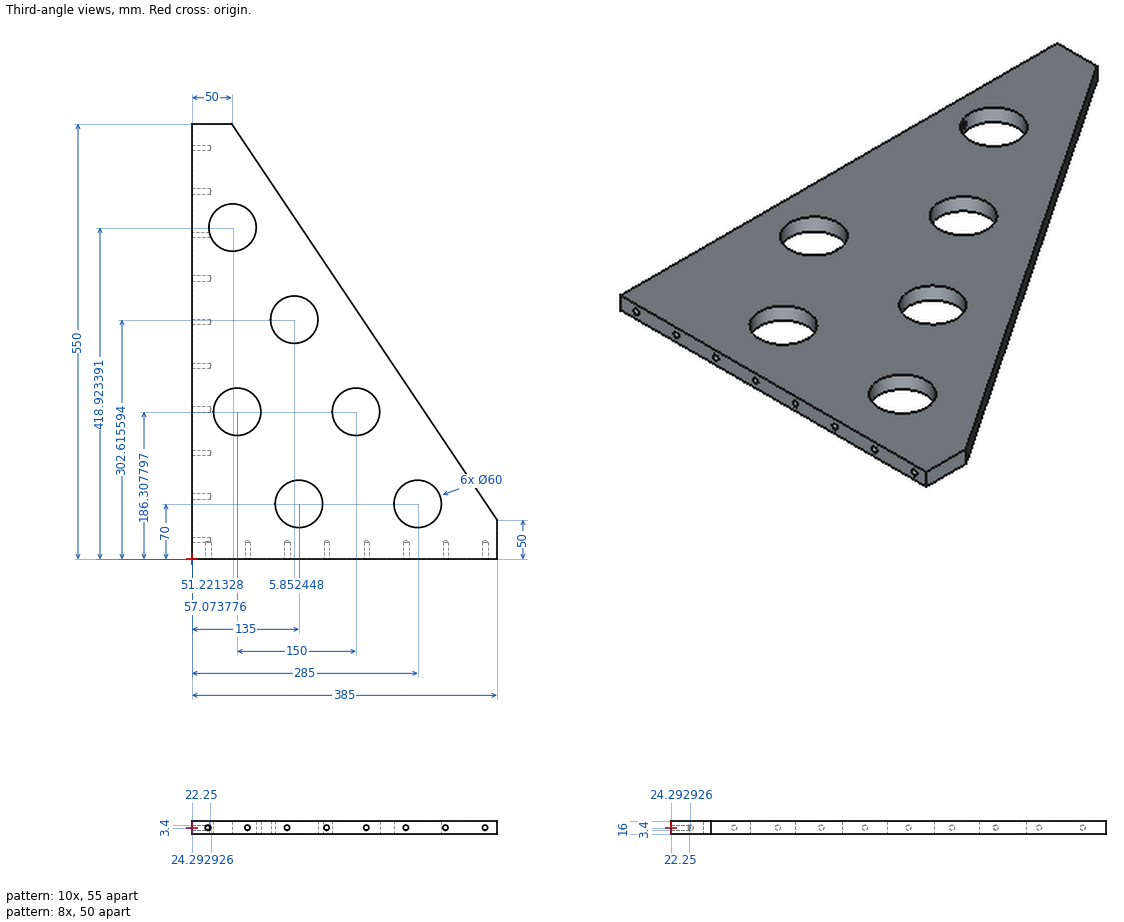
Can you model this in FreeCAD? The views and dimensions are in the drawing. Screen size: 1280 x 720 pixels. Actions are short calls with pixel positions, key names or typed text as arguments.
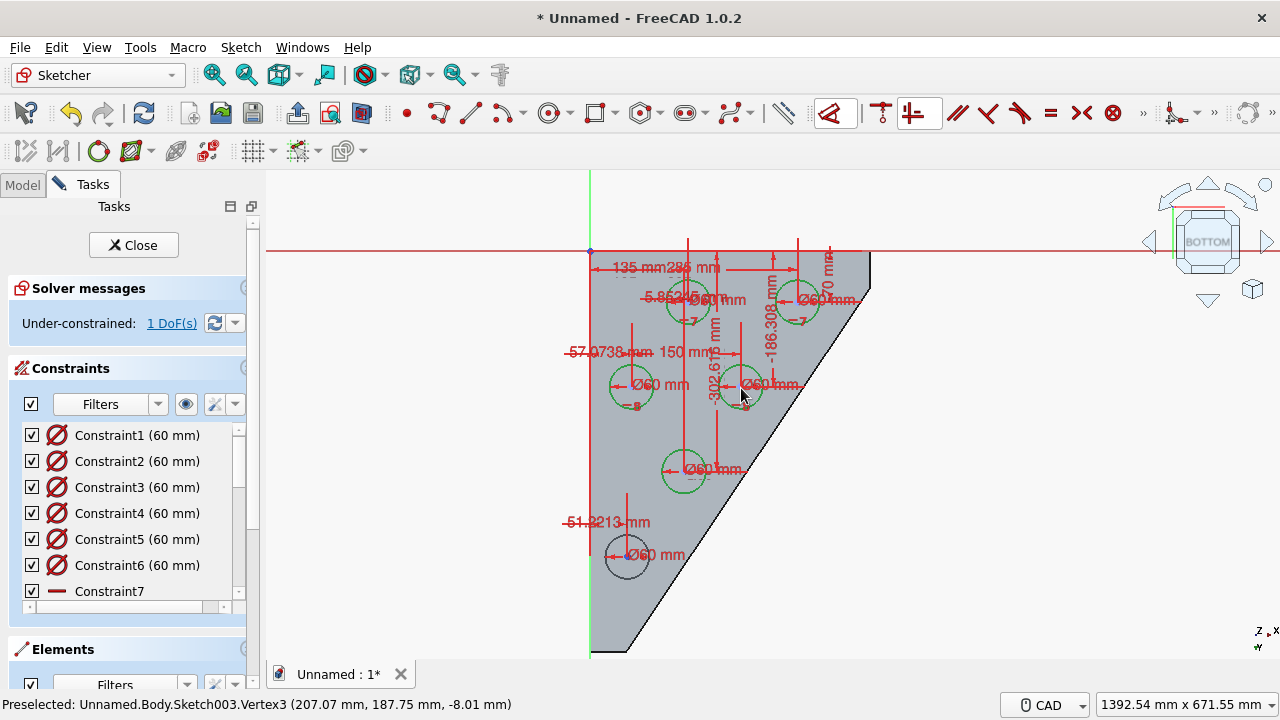
click(627, 557)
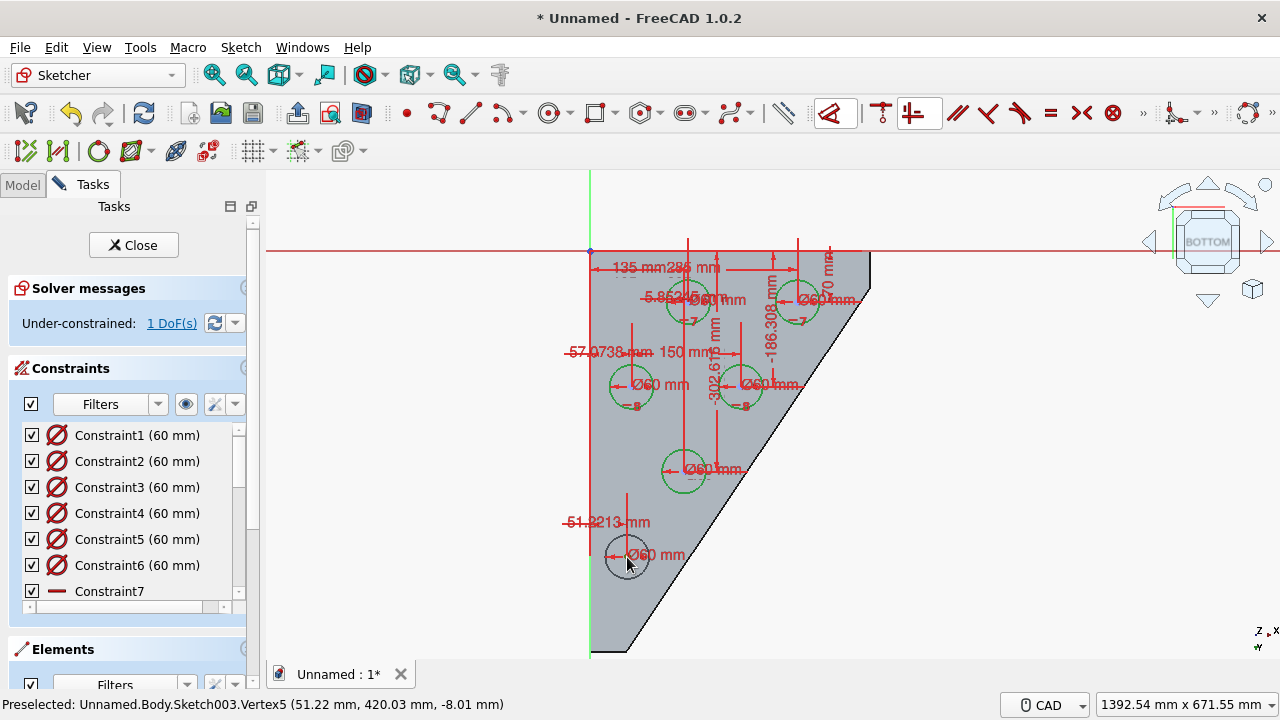
key(i)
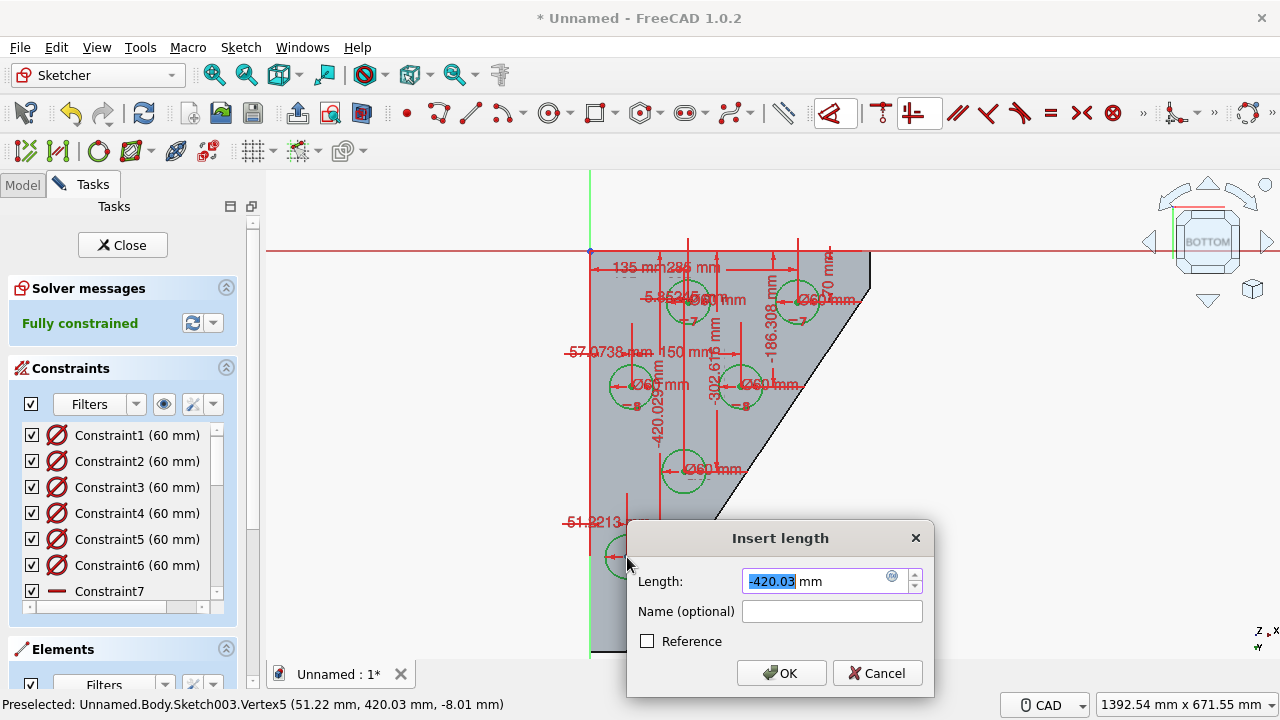
text(-418.923391)
key(Return)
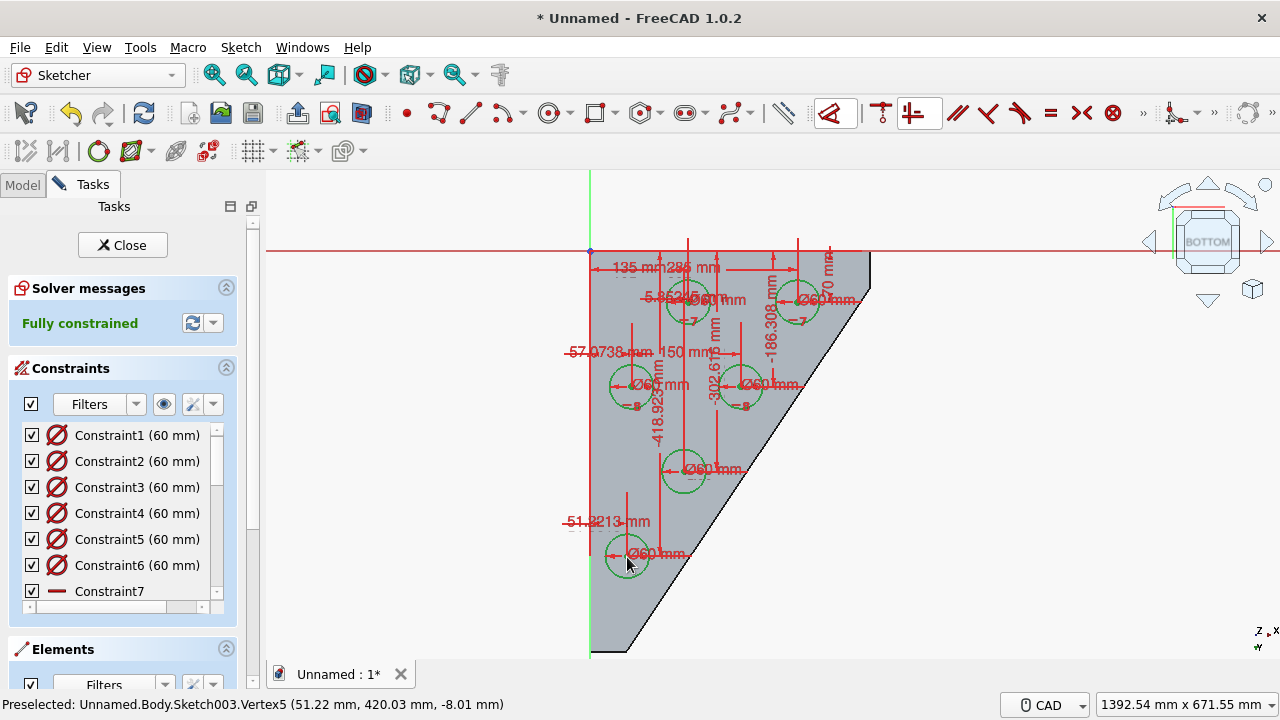
click(123, 245)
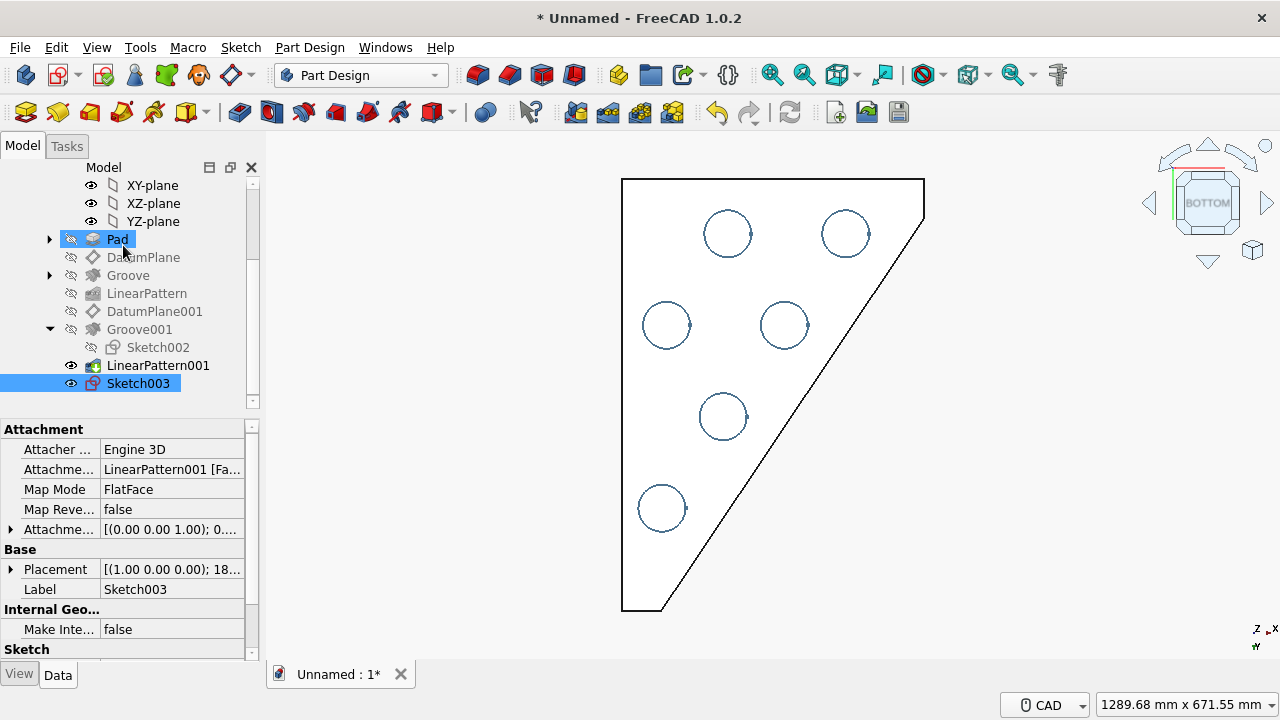
click(240, 112)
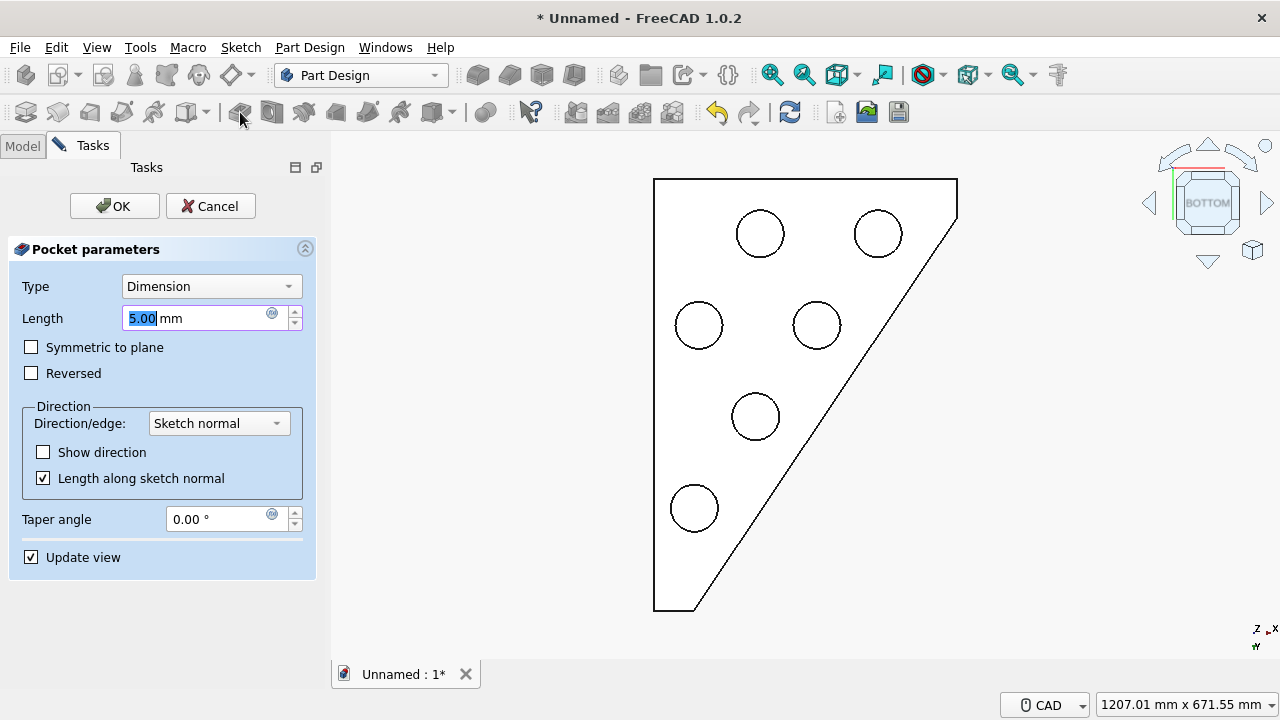
click(212, 286)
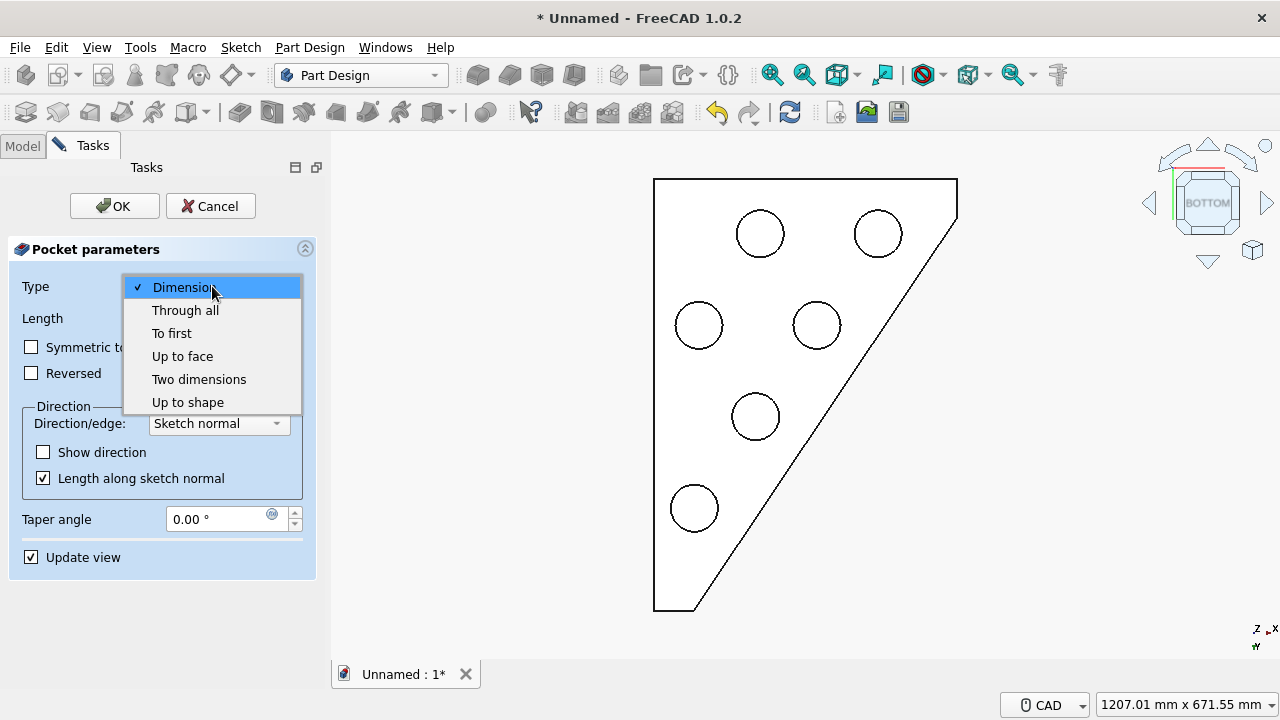
click(212, 310)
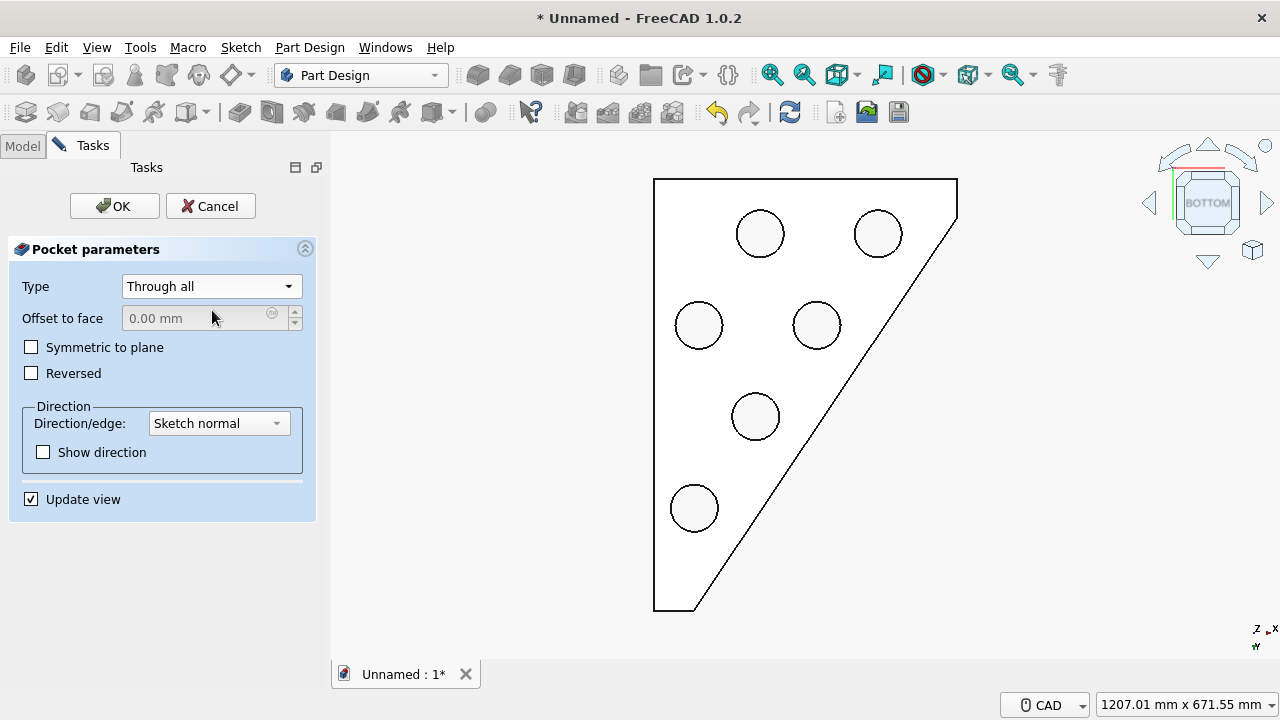
click(115, 206)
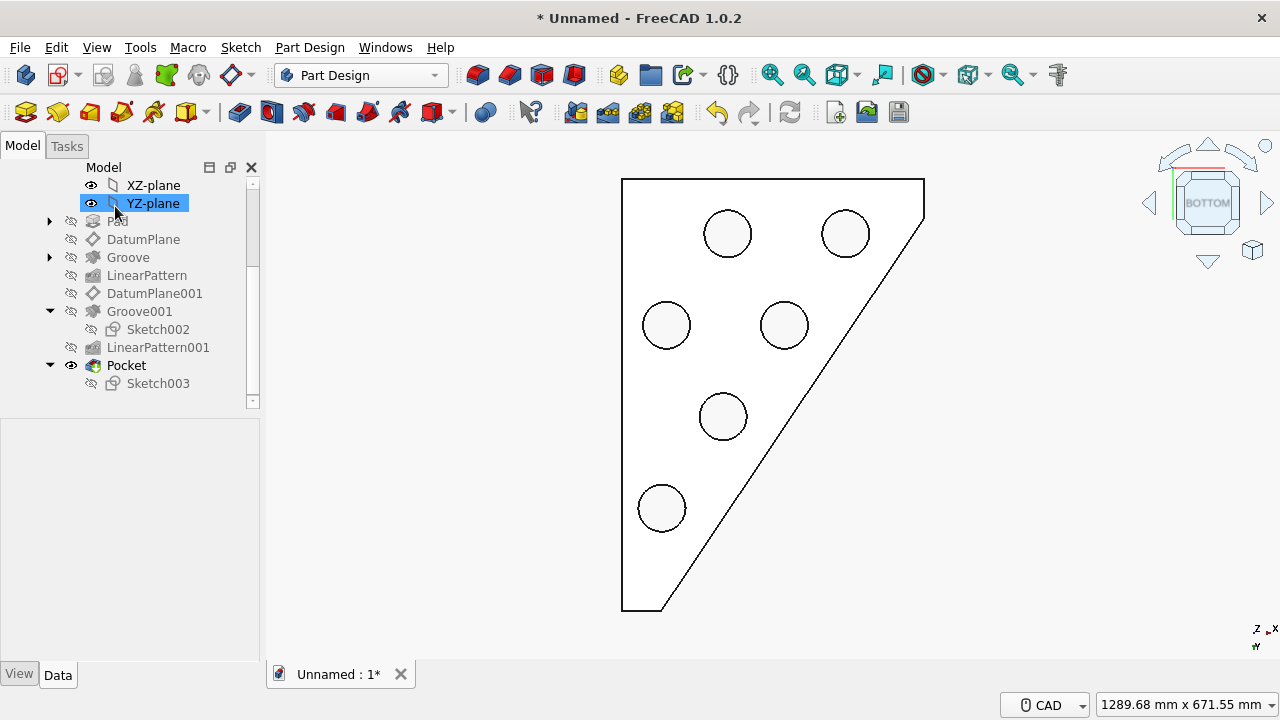
key(0)